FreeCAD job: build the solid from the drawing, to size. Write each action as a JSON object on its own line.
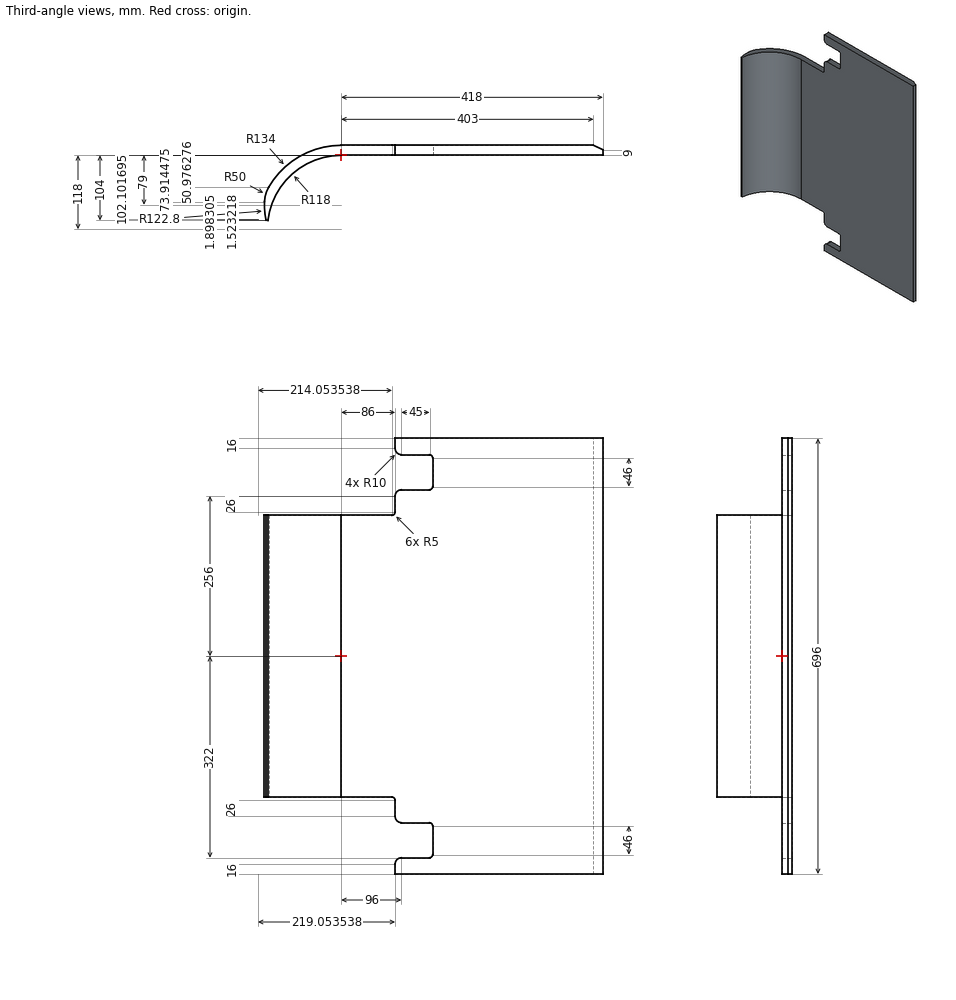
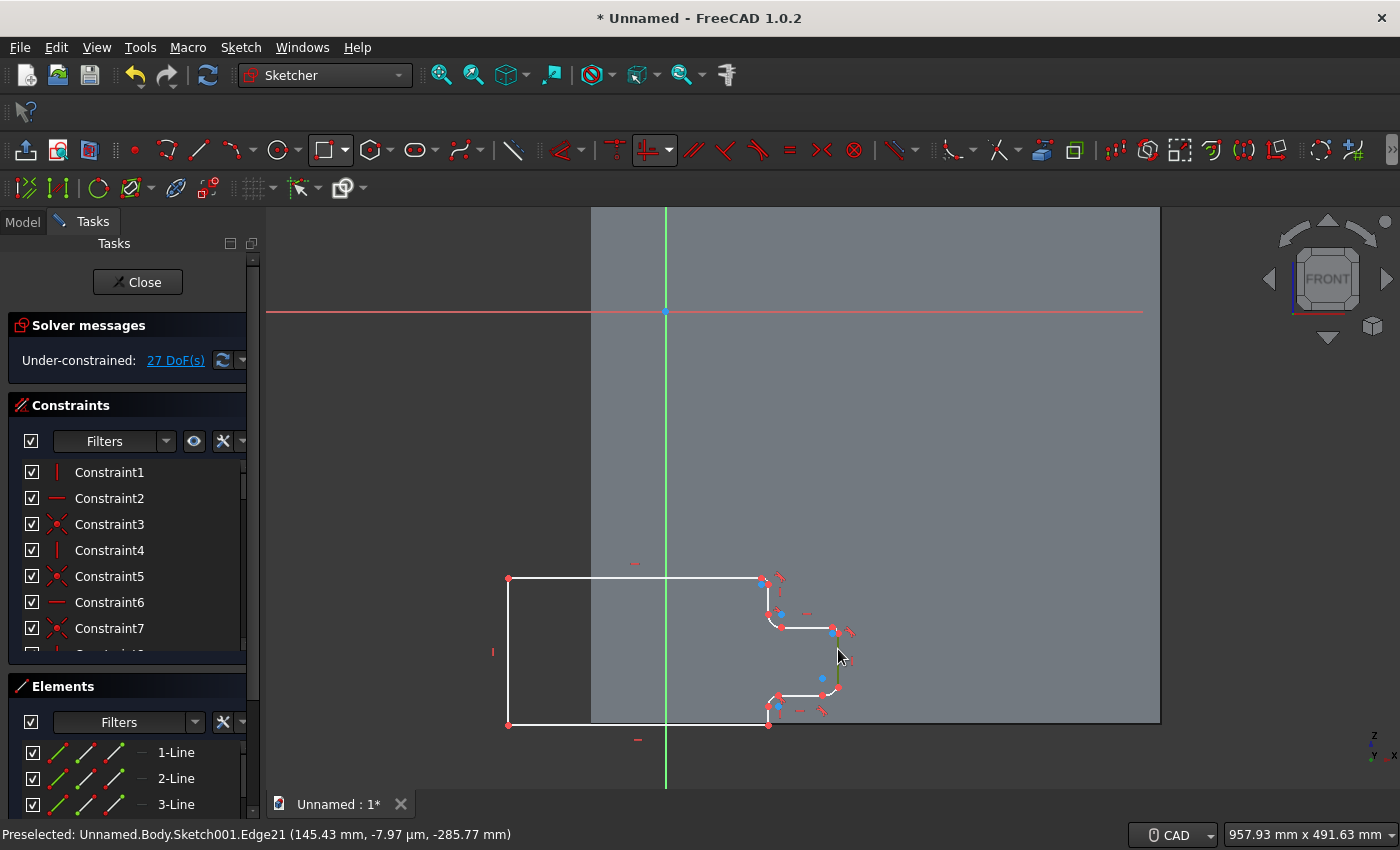
{"action": "scroll", "coordinate": [832, 694], "scroll_direction": "up", "scroll_amount": 3}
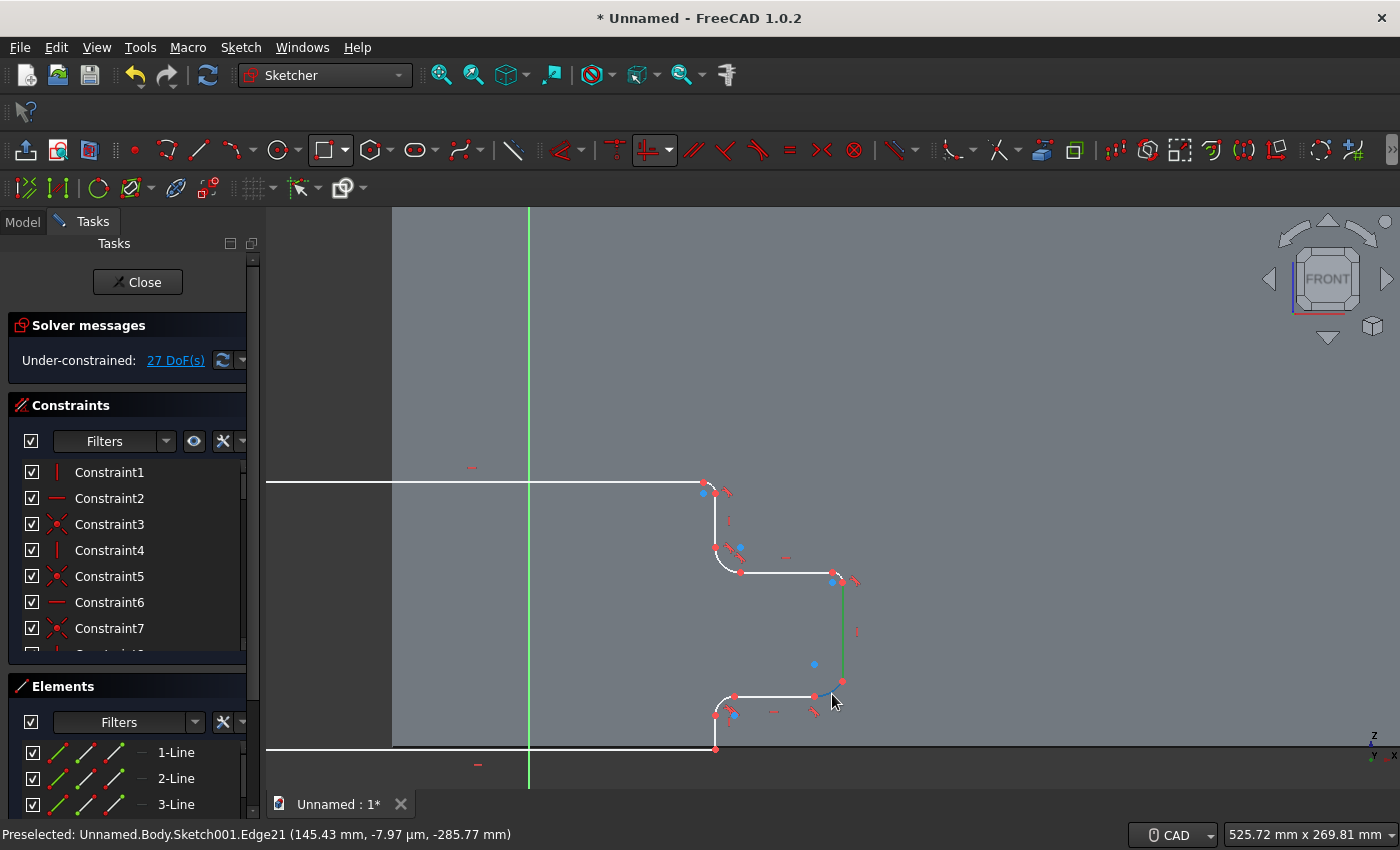
{"action": "left_click", "coordinate": [831, 692]}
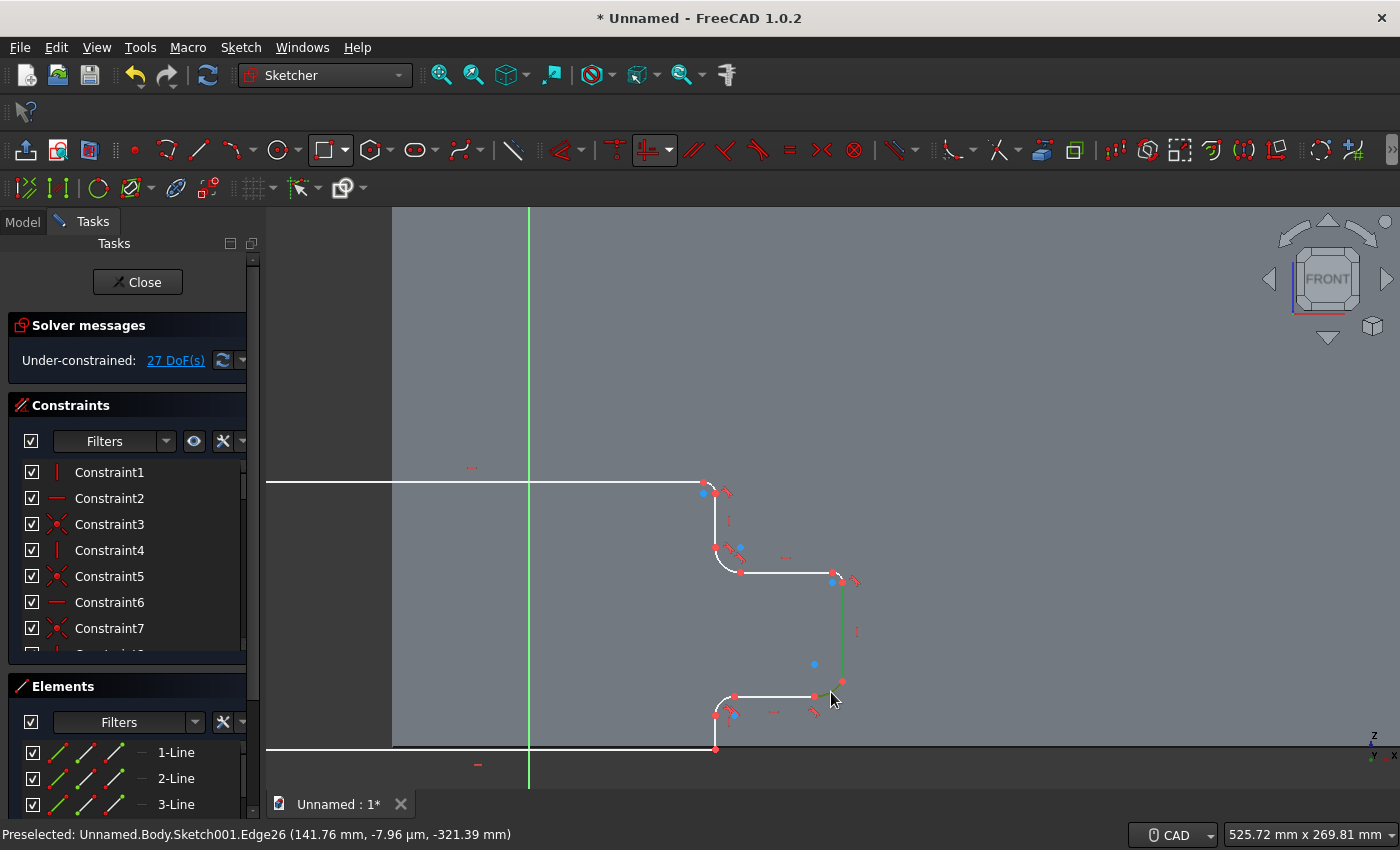
{"action": "left_click", "coordinate": [758, 150]}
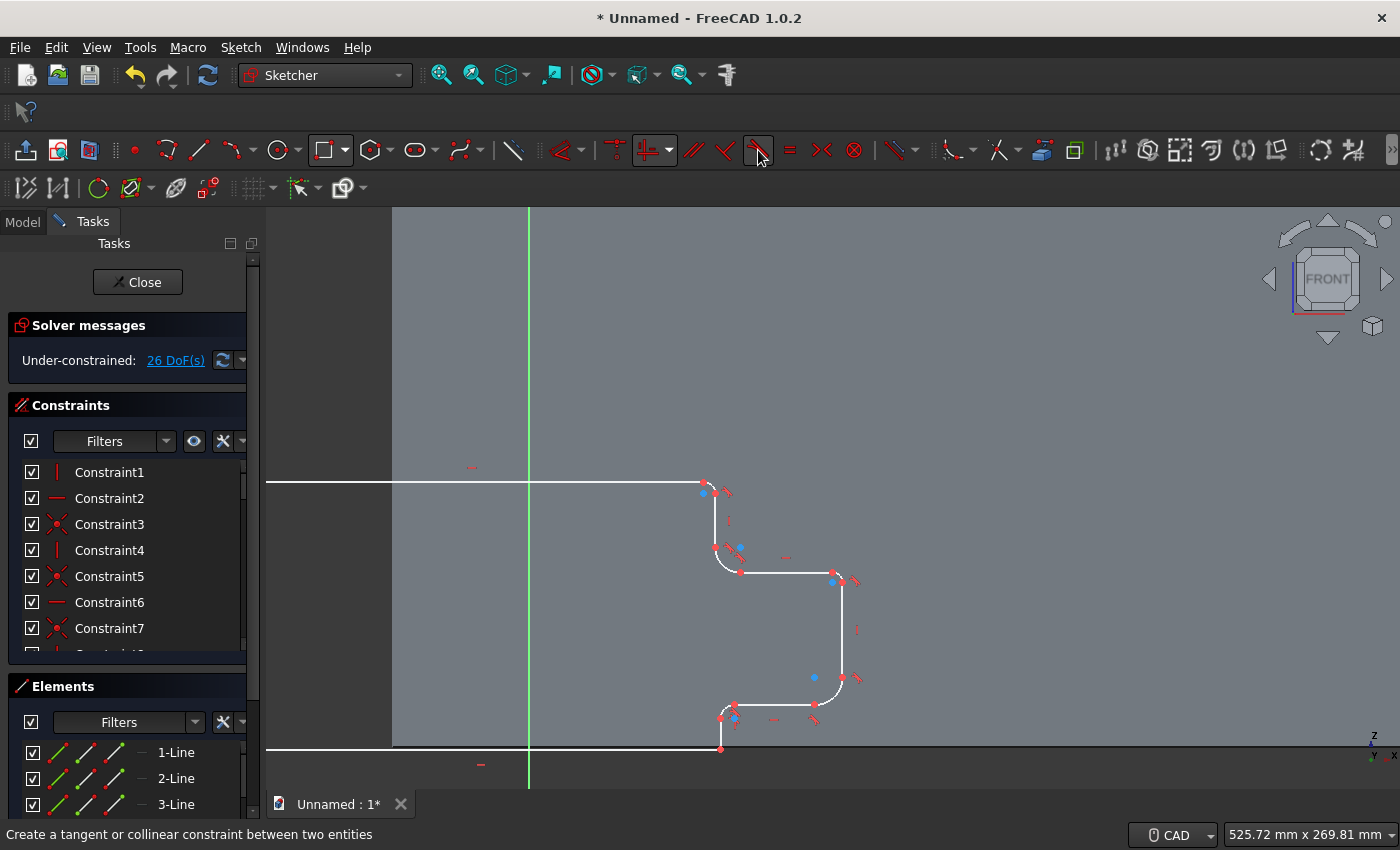
{"action": "scroll", "coordinate": [837, 662], "scroll_direction": "down", "scroll_amount": 7}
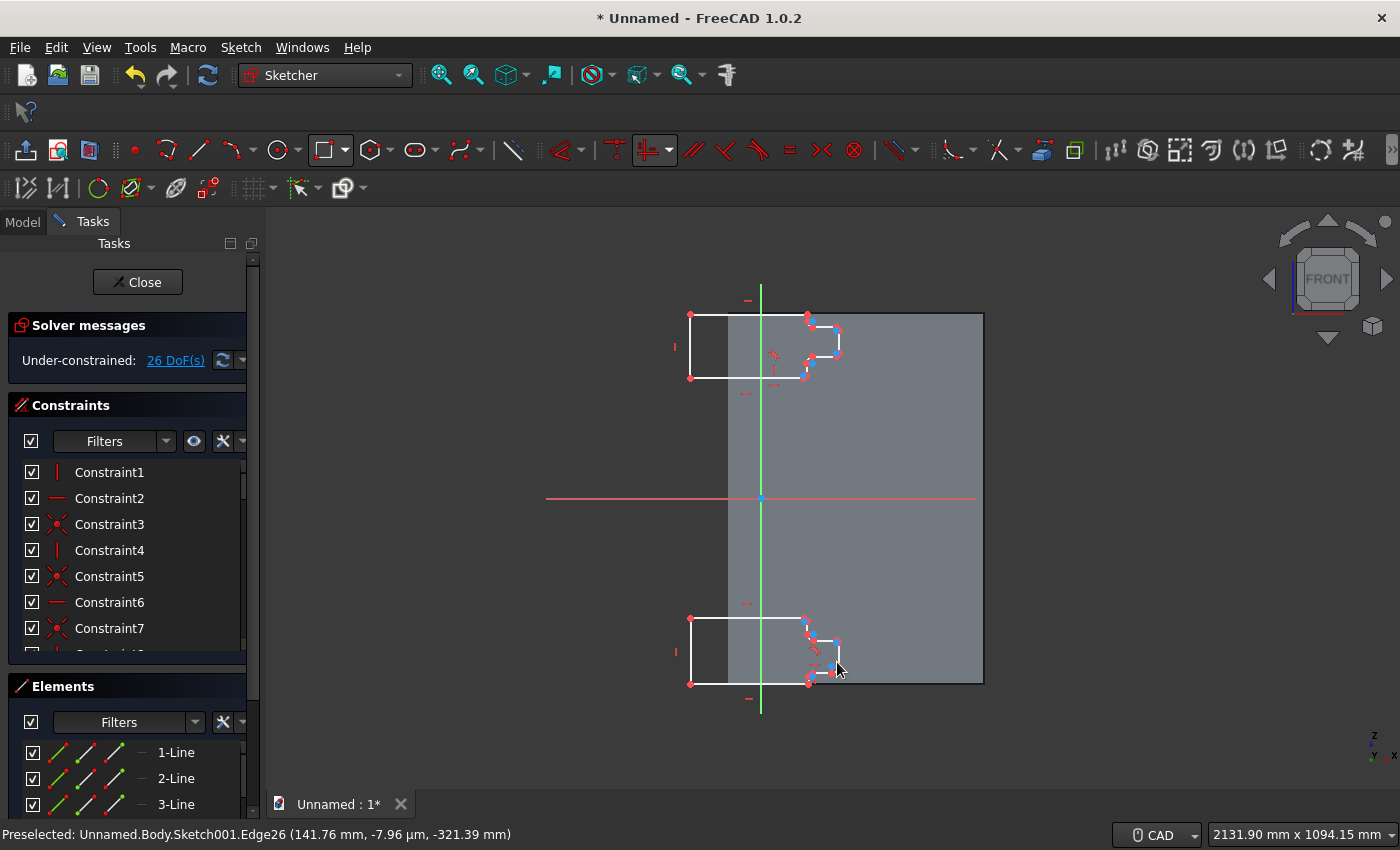
{"action": "scroll", "coordinate": [806, 378], "scroll_direction": "up", "scroll_amount": 10}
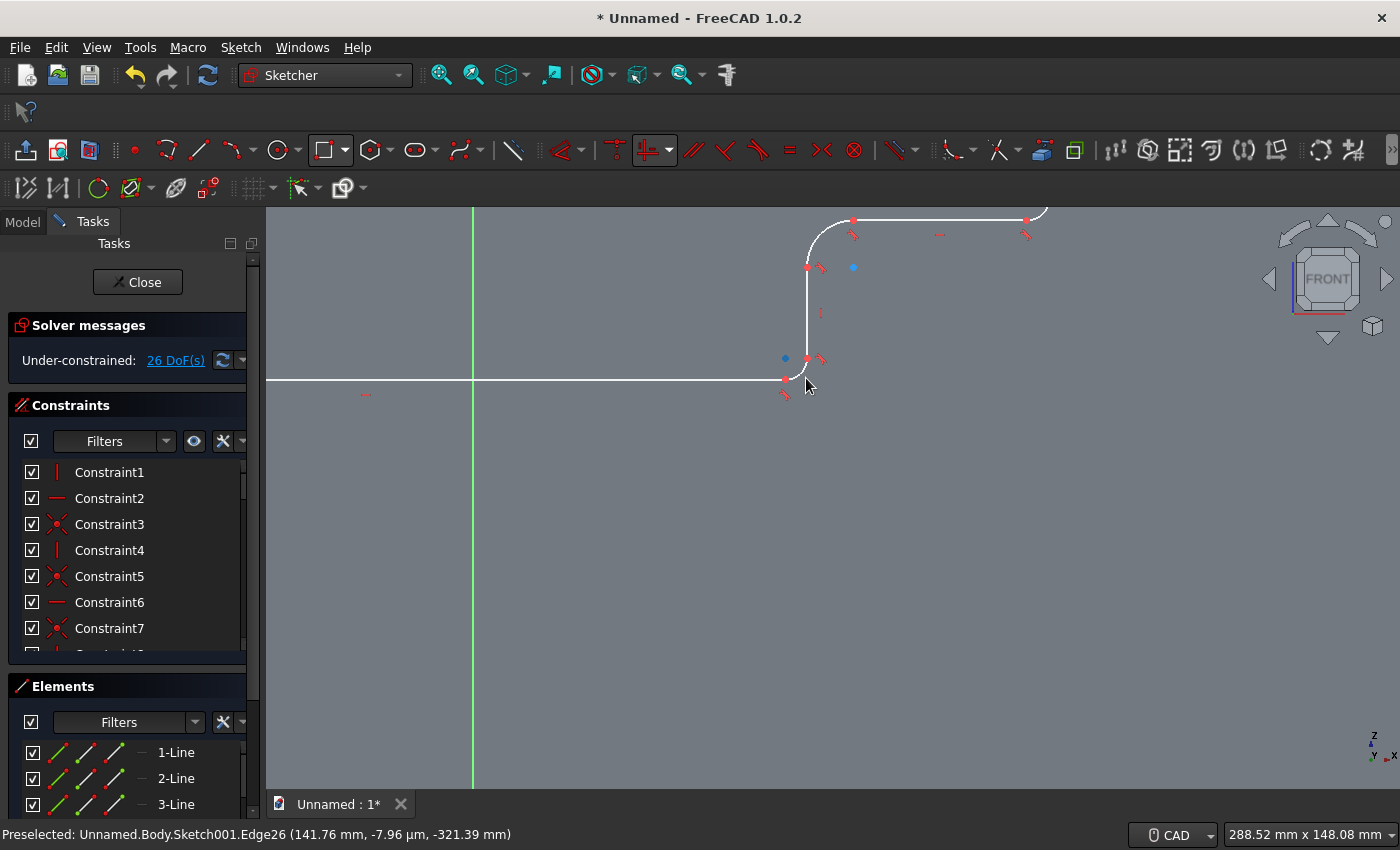
{"action": "left_click", "coordinate": [801, 373]}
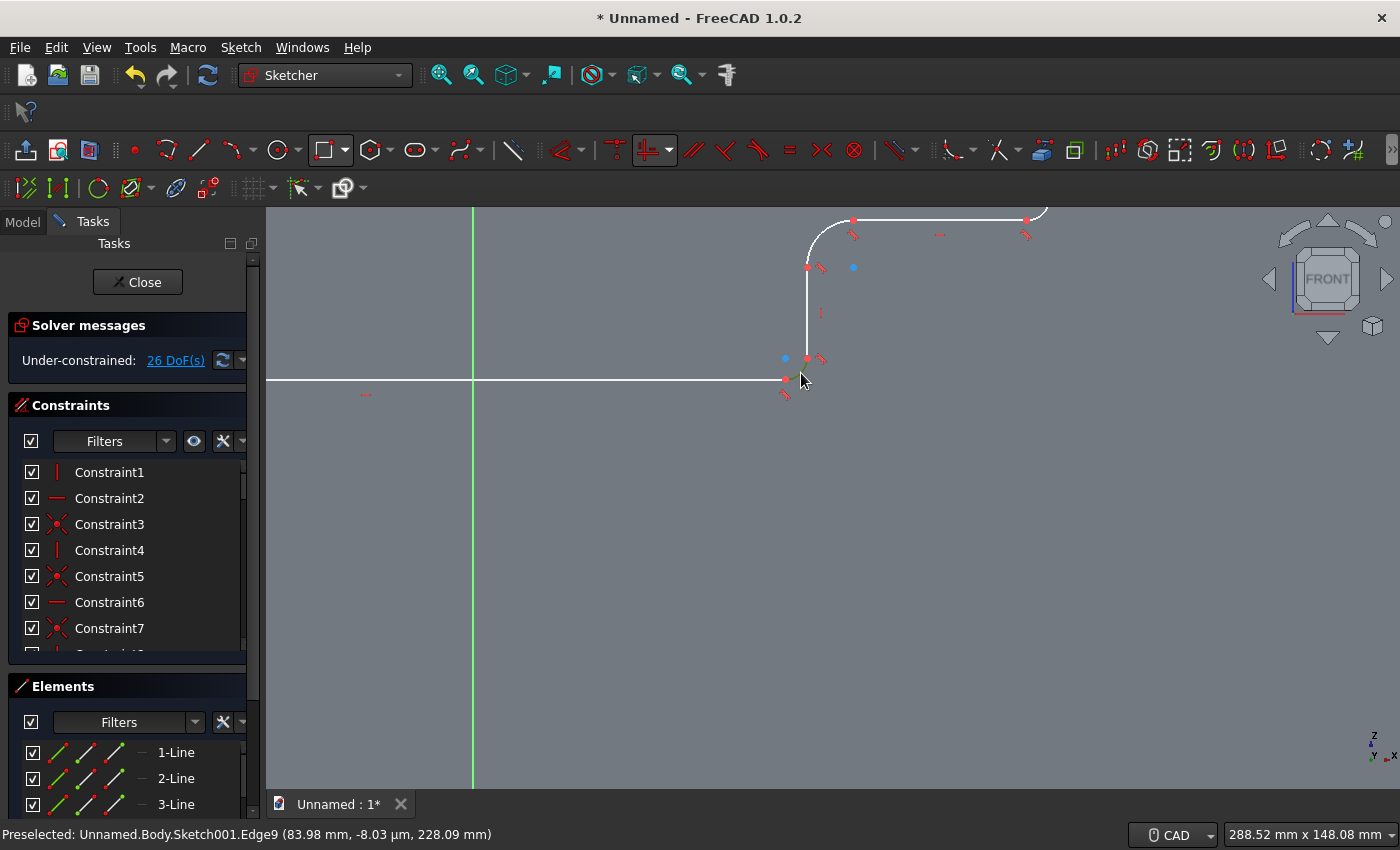
{"action": "scroll", "coordinate": [806, 378], "scroll_direction": "down", "scroll_amount": 10}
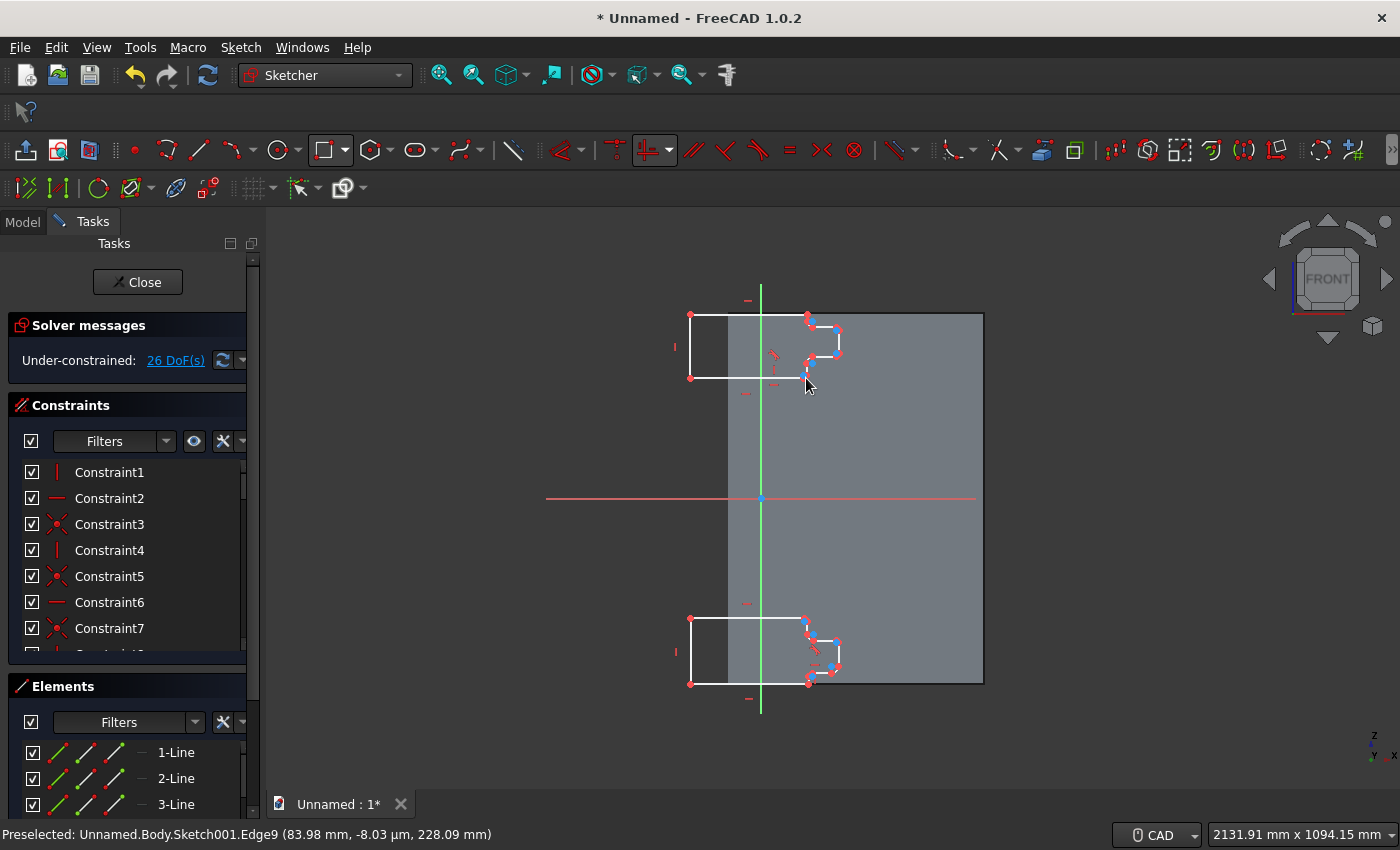
{"action": "scroll", "coordinate": [839, 329], "scroll_direction": "up", "scroll_amount": 12}